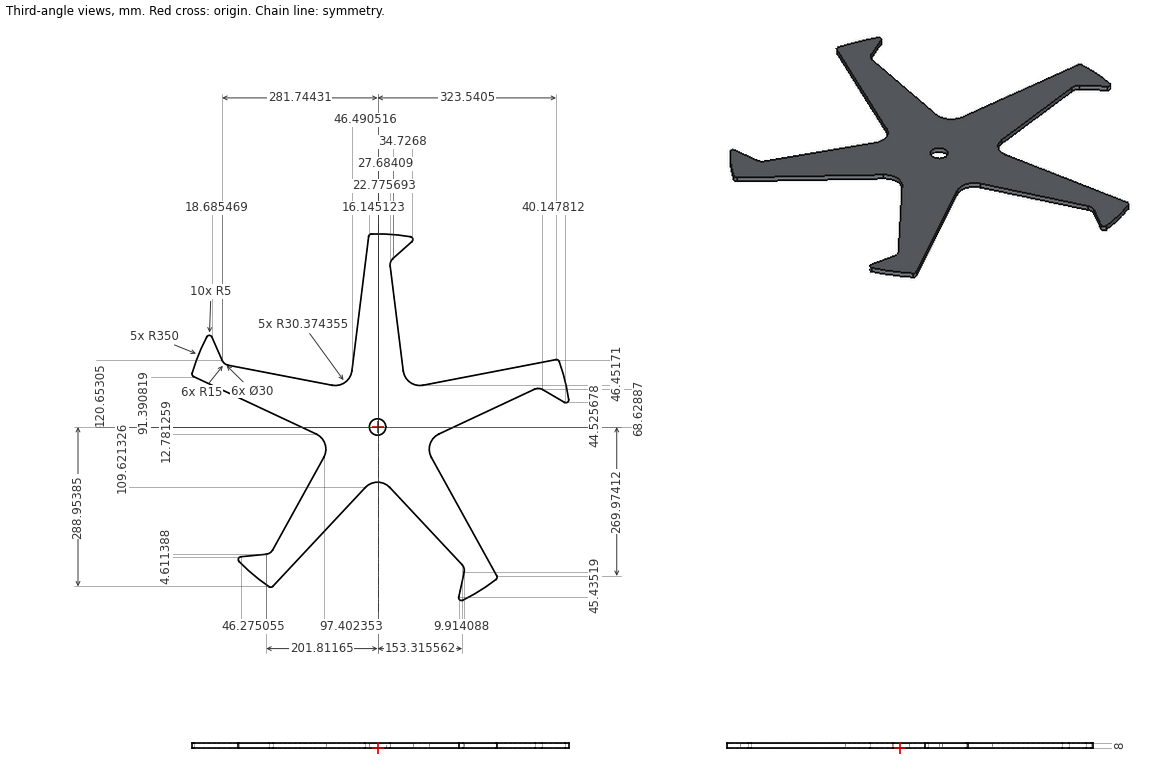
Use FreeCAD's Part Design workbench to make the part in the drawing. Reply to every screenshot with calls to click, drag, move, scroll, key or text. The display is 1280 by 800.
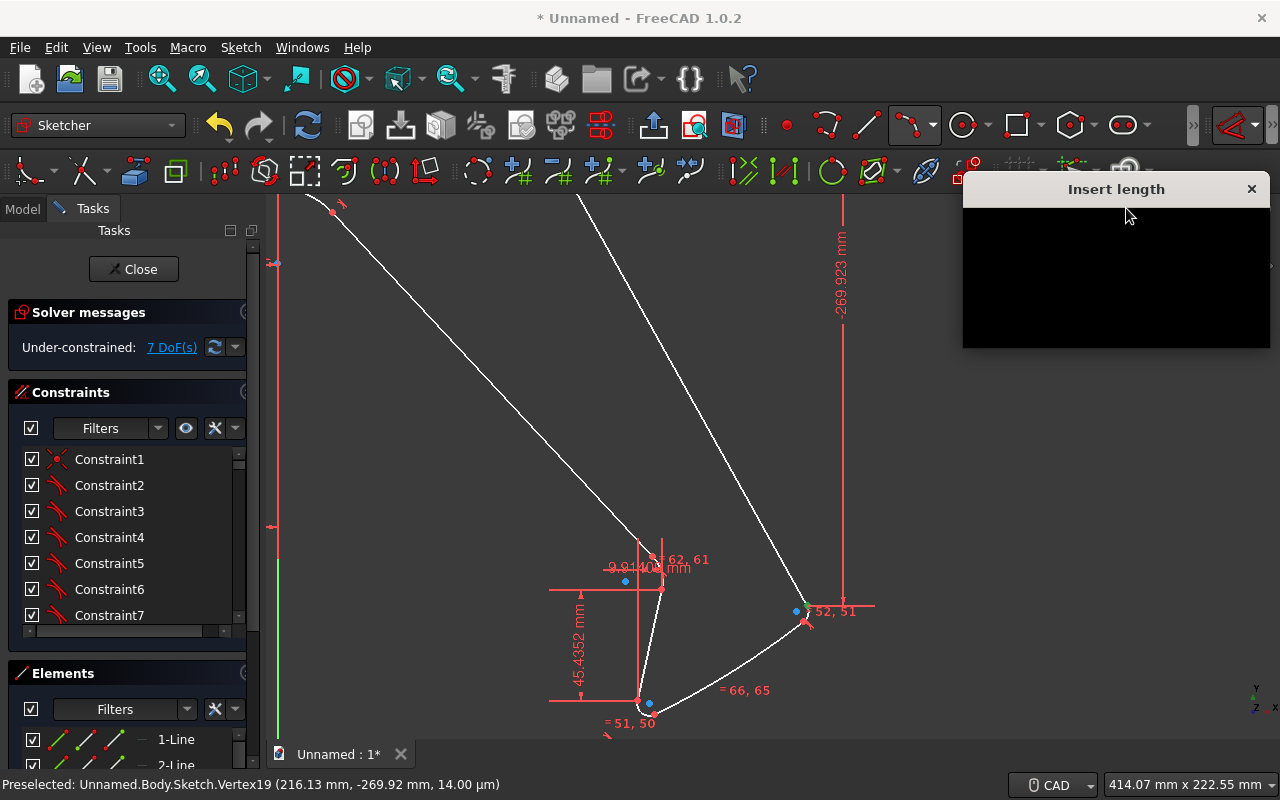
text(-269.97412)
key(Return)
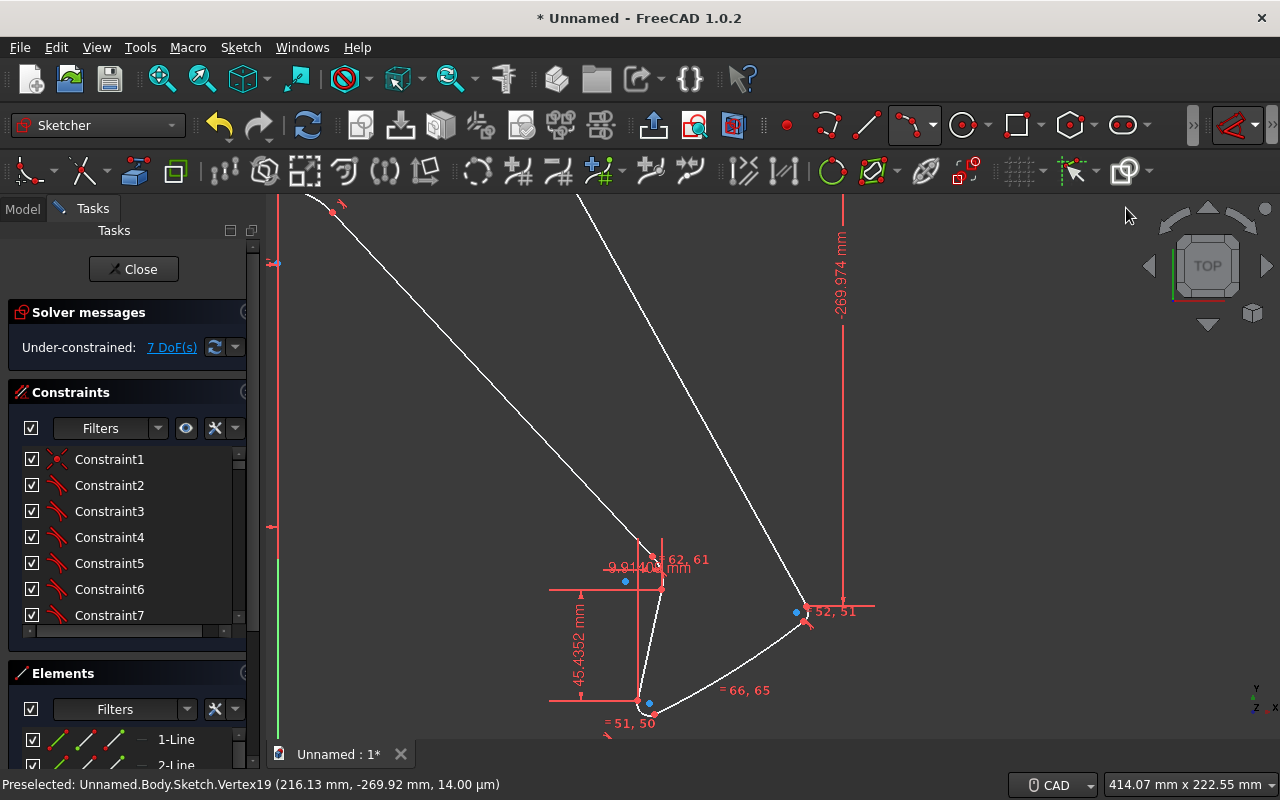
scroll(809, 609, down, 8)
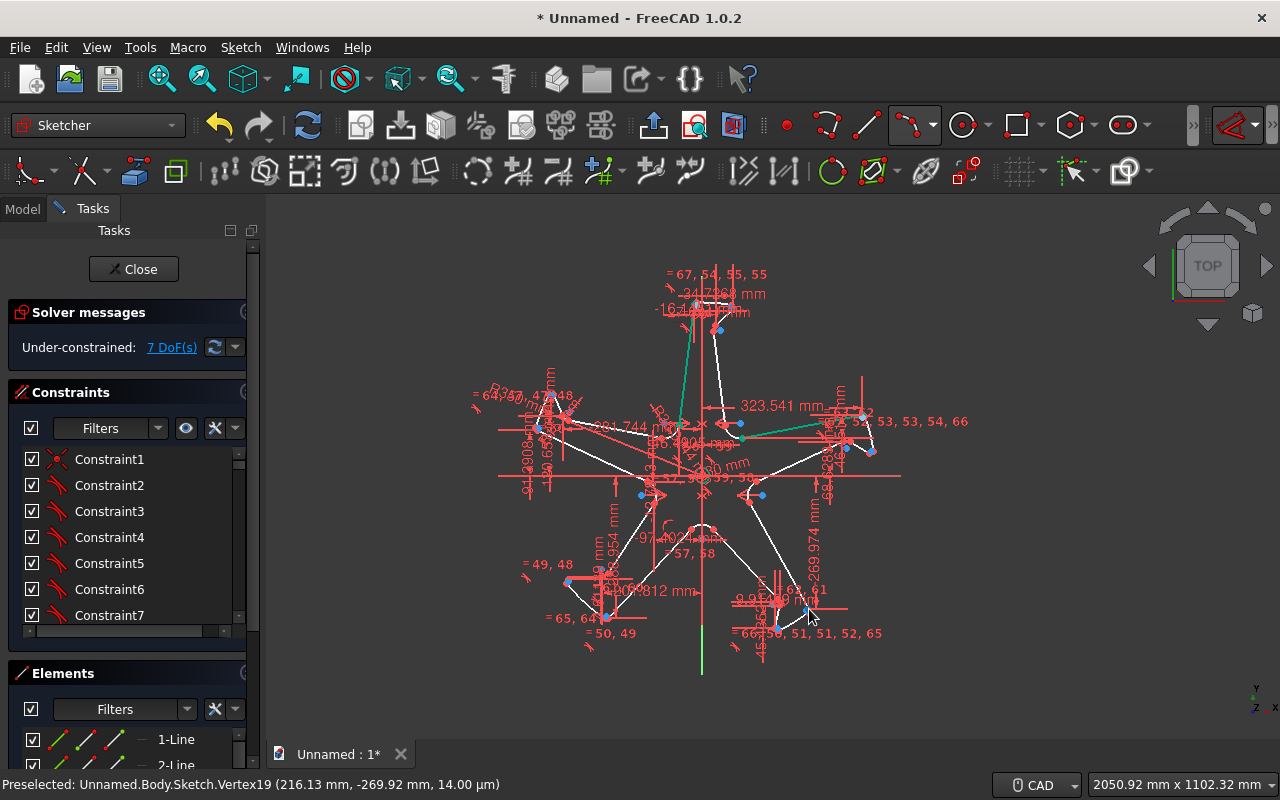
scroll(870, 454, up, 8)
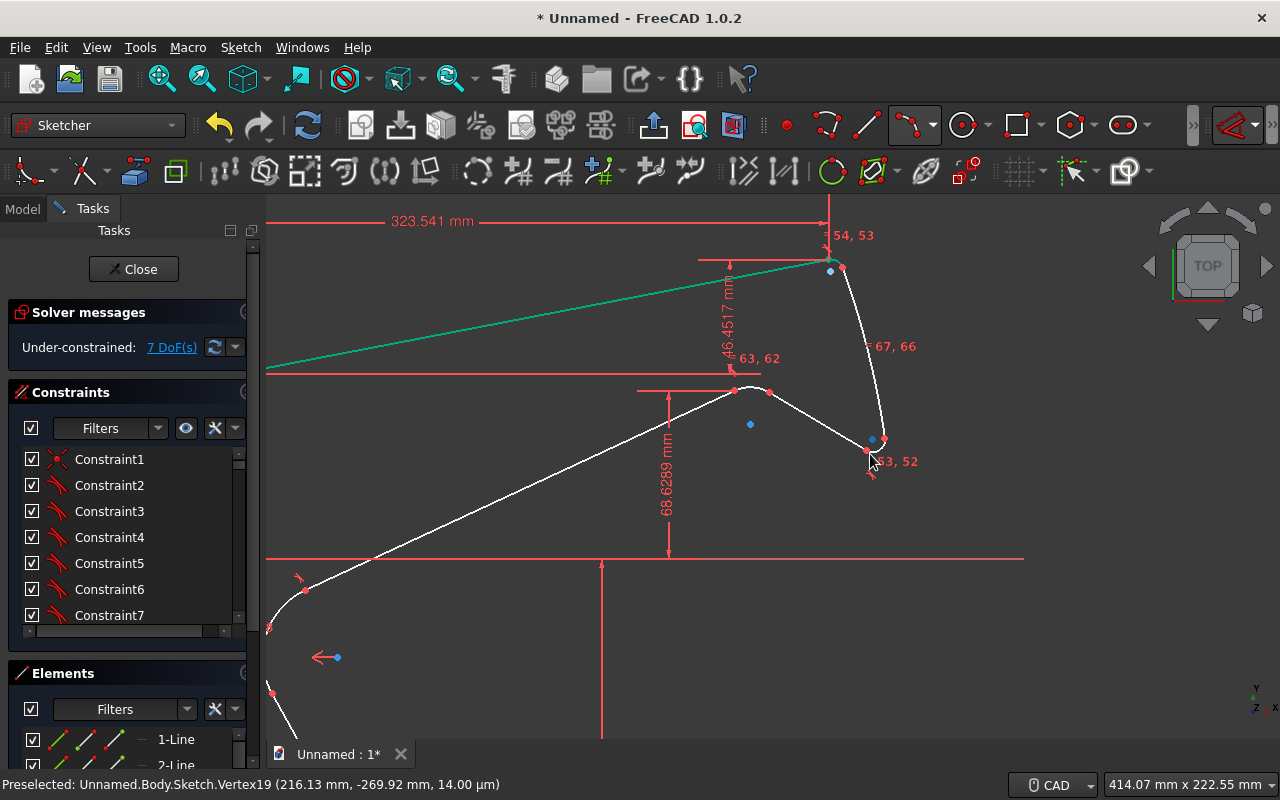
click(867, 450)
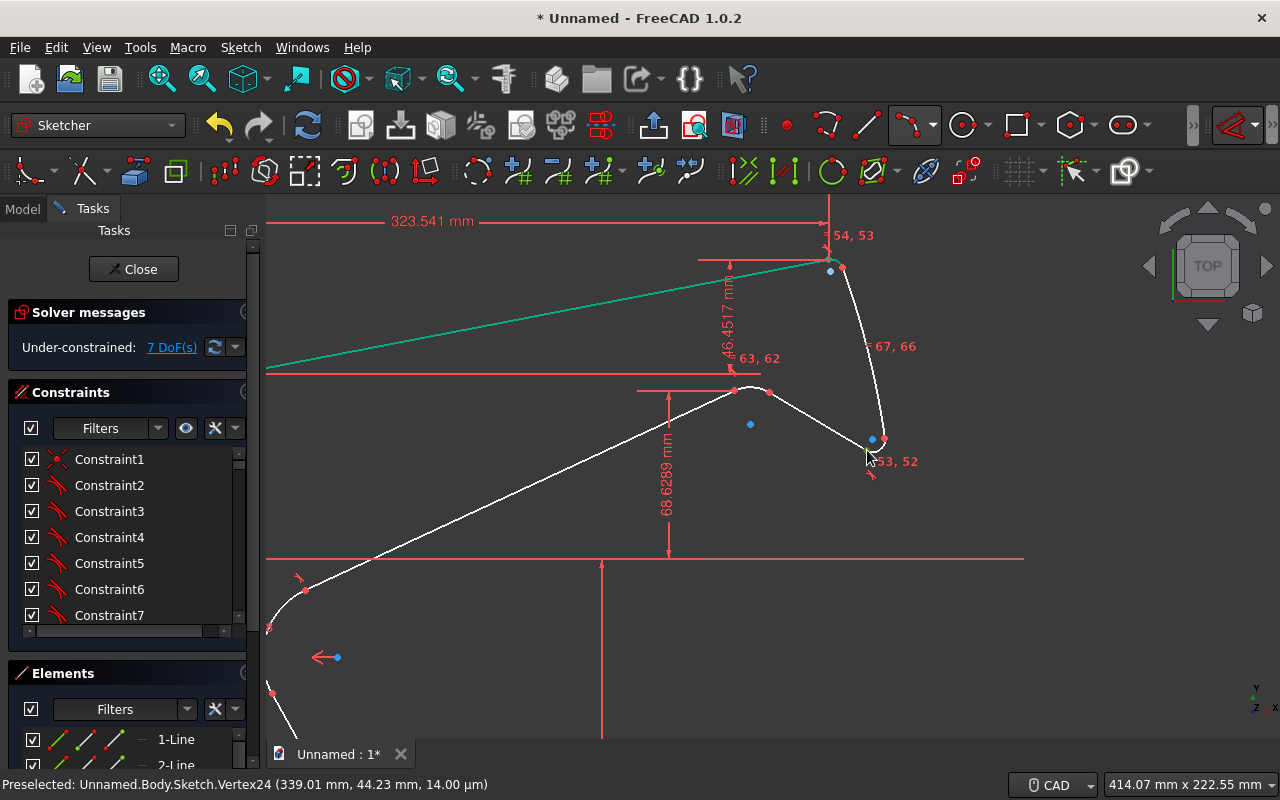
click(1258, 126)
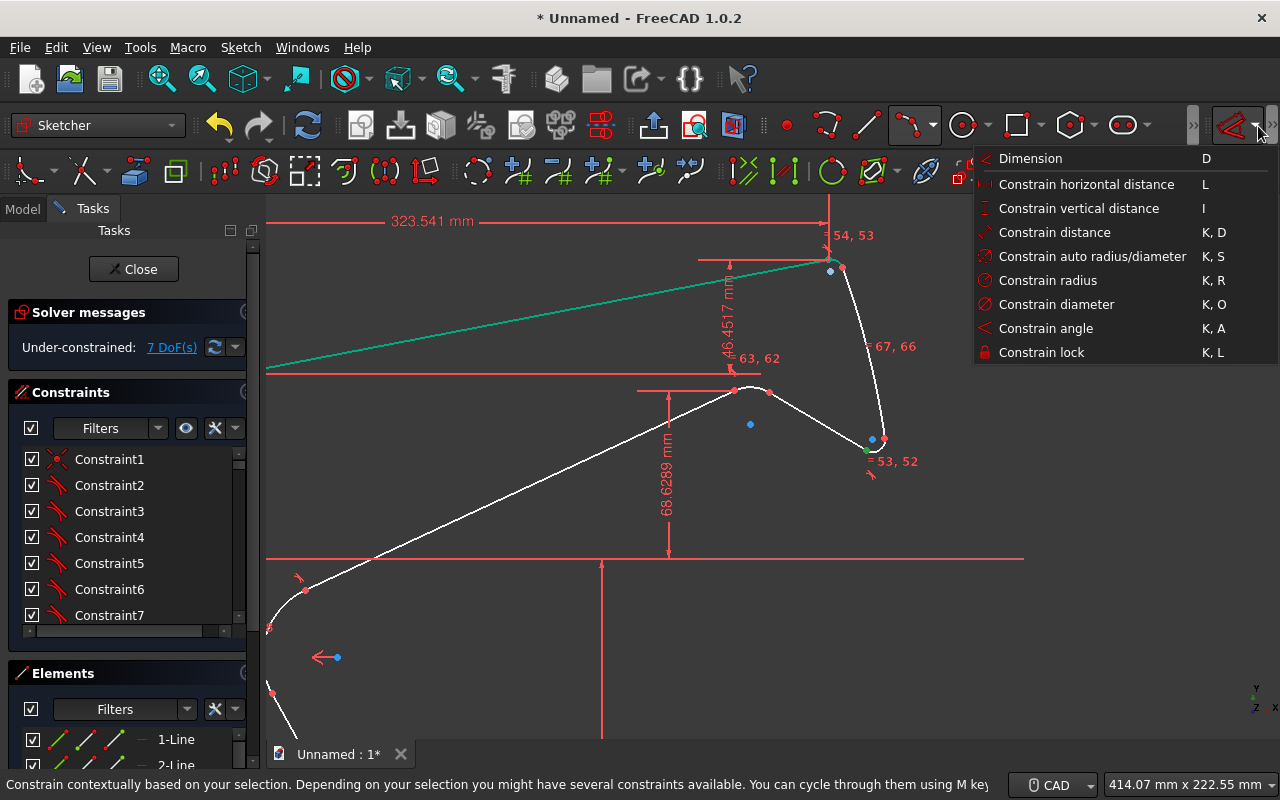
click(1126, 208)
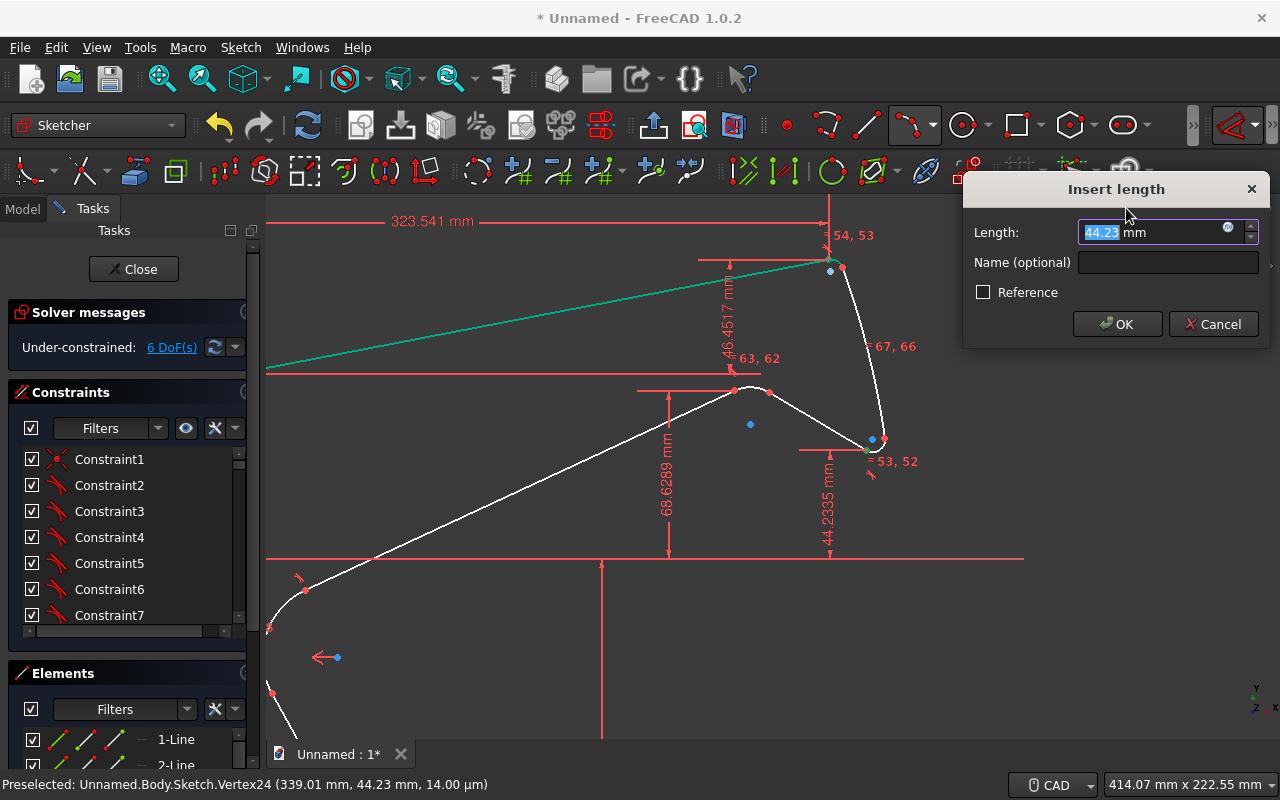
text(44.525678)
key(Return)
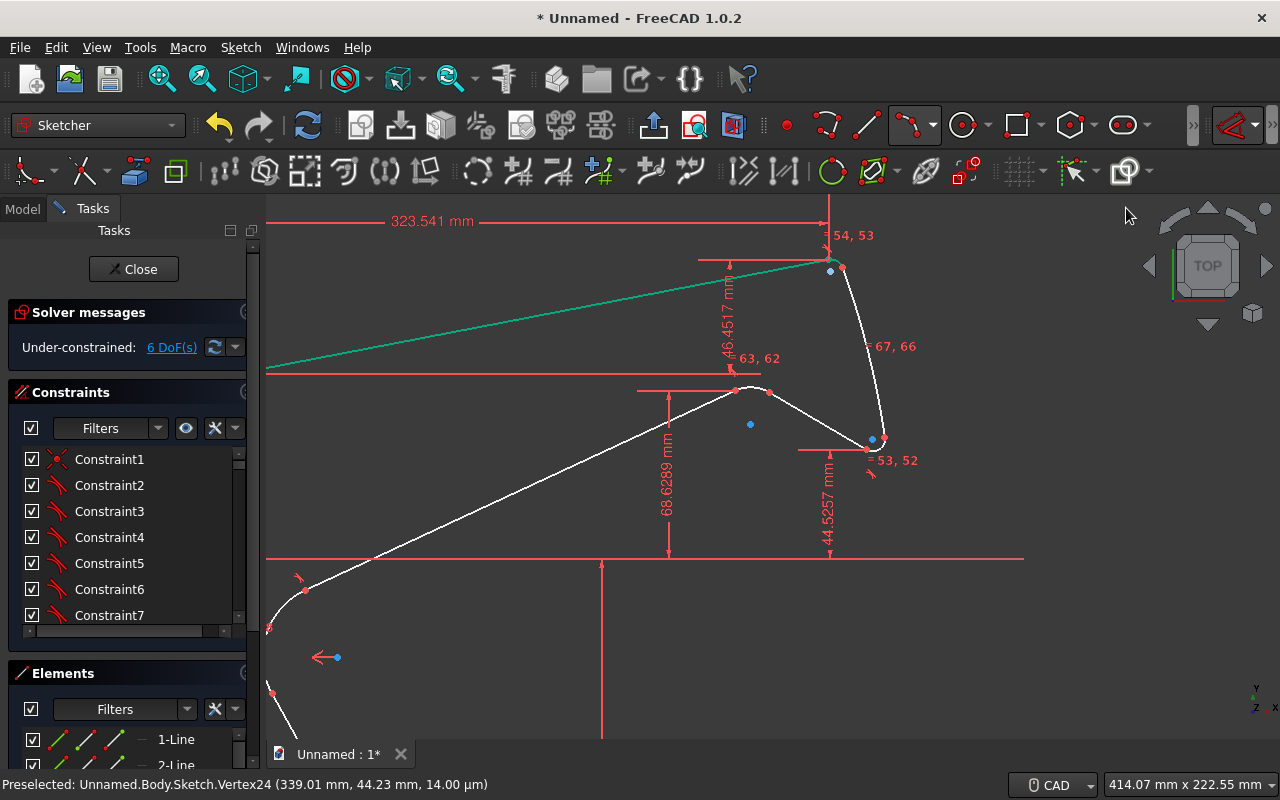
scroll(870, 454, down, 8)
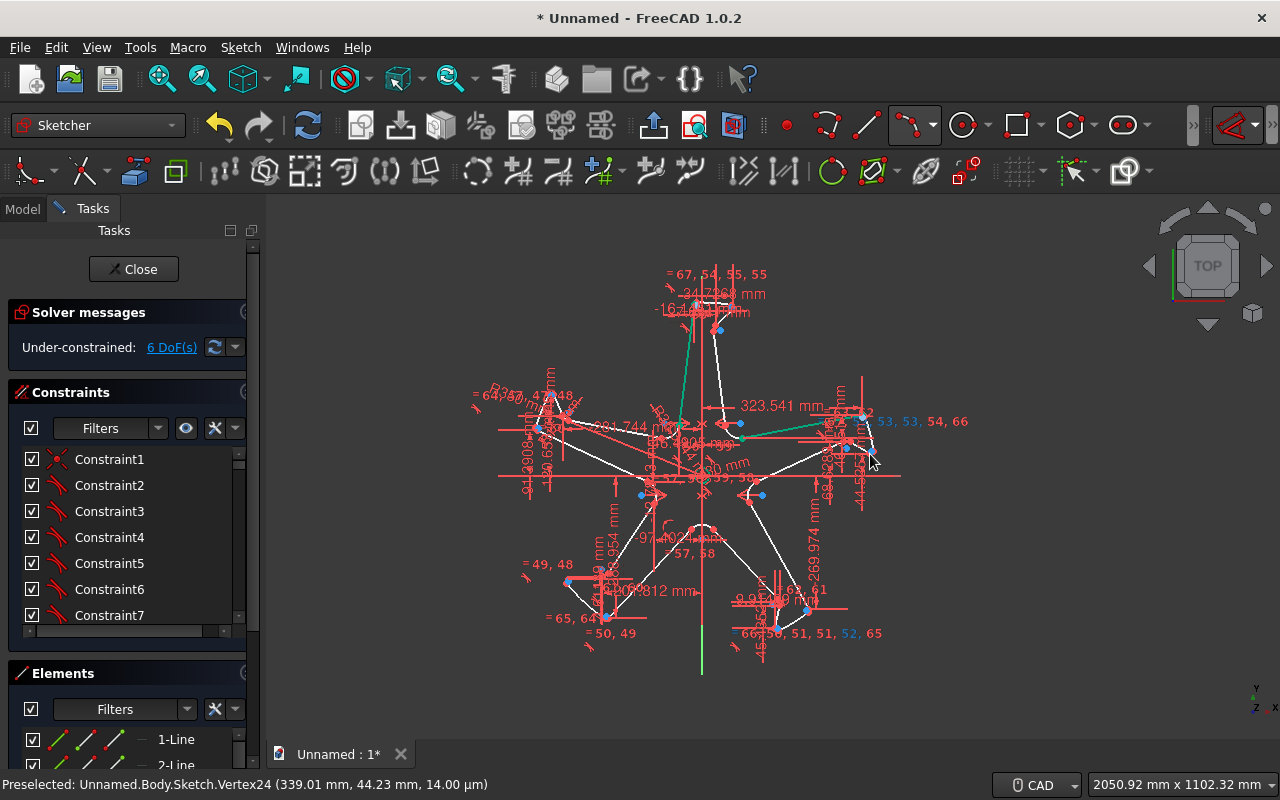
scroll(714, 332, up, 7)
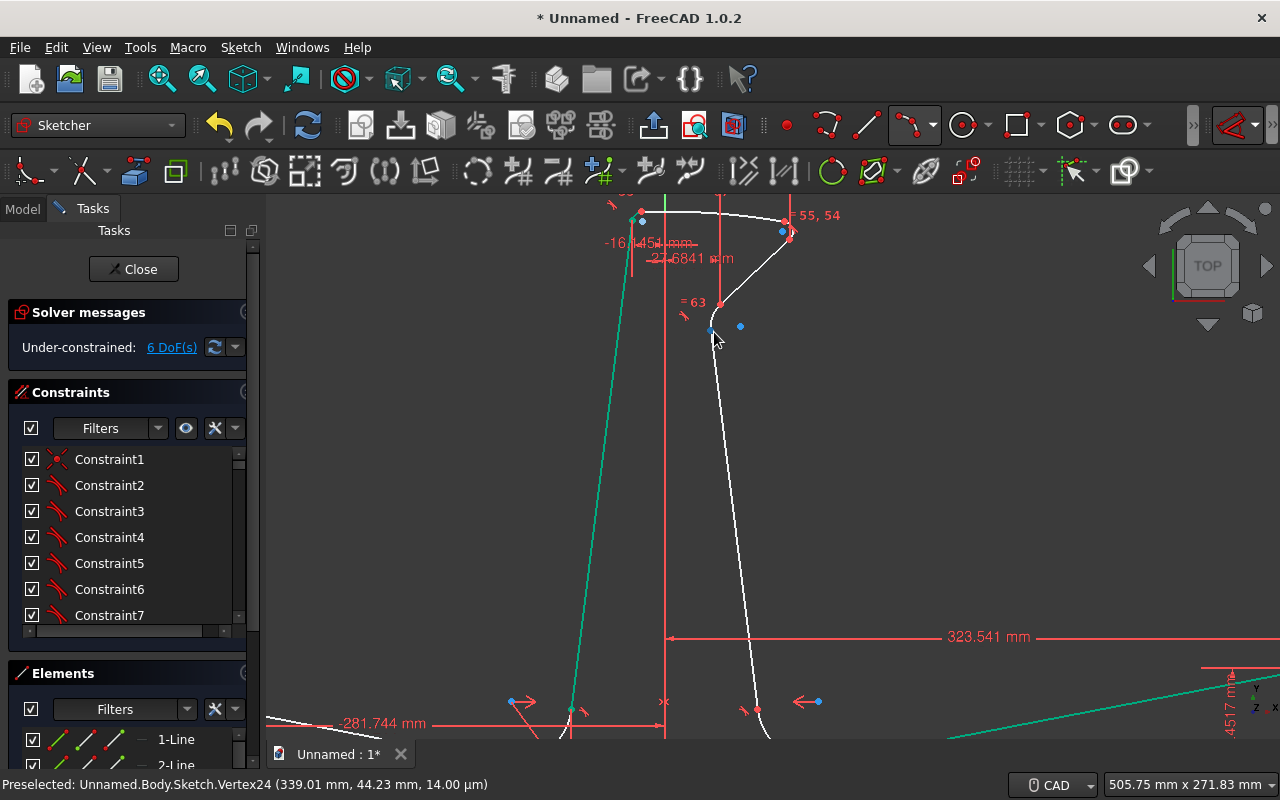
click(711, 330)